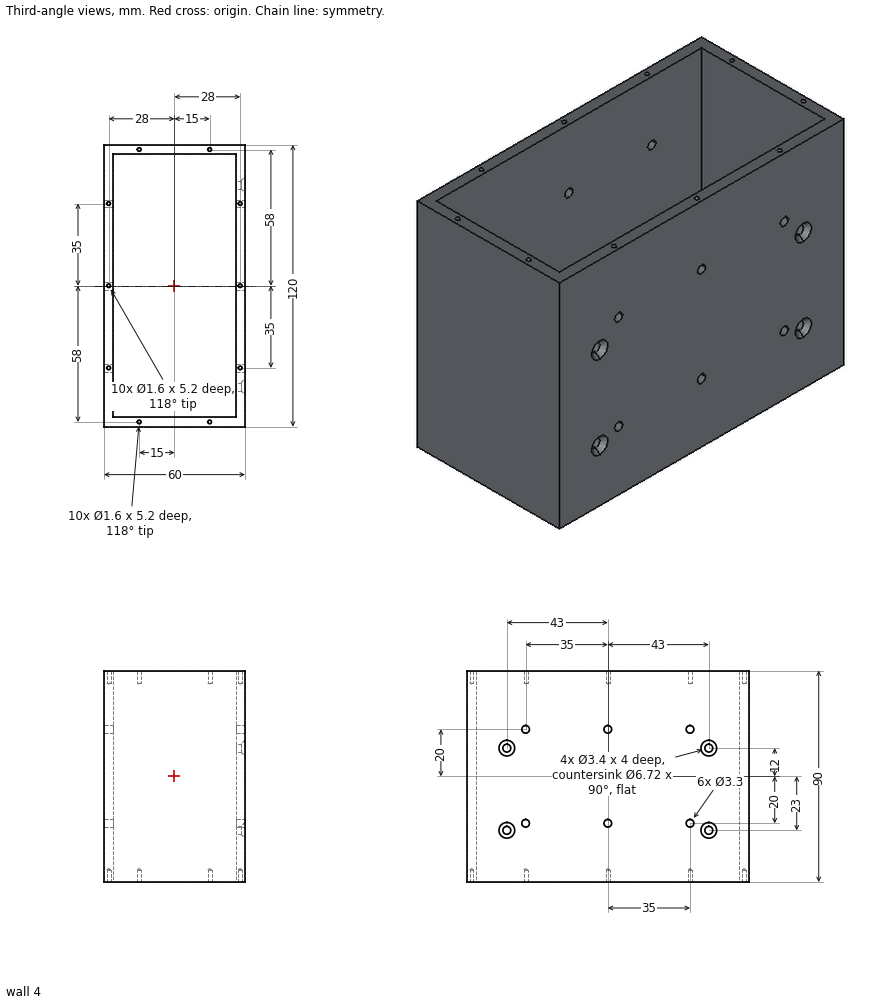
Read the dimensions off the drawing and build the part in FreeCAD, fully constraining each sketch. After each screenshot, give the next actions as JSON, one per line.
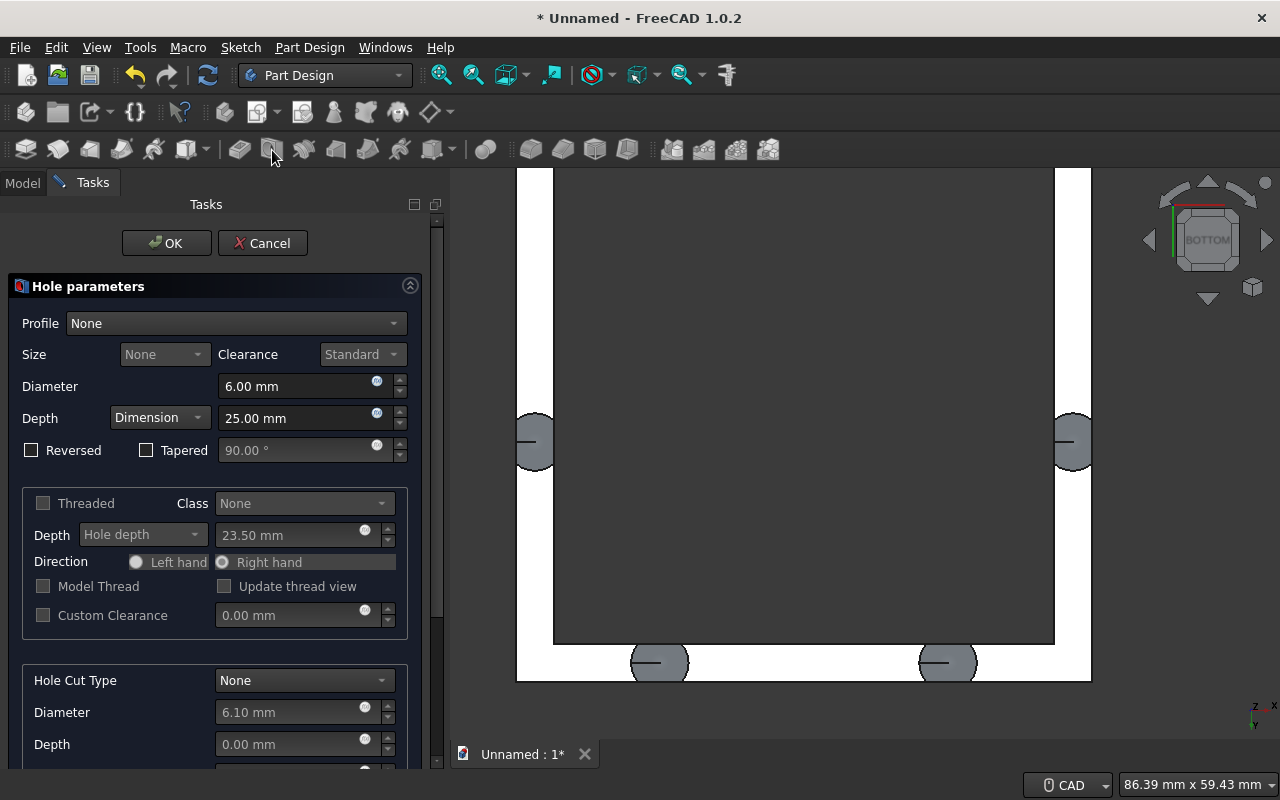
{"action": "triple_click", "coordinate": [305, 386]}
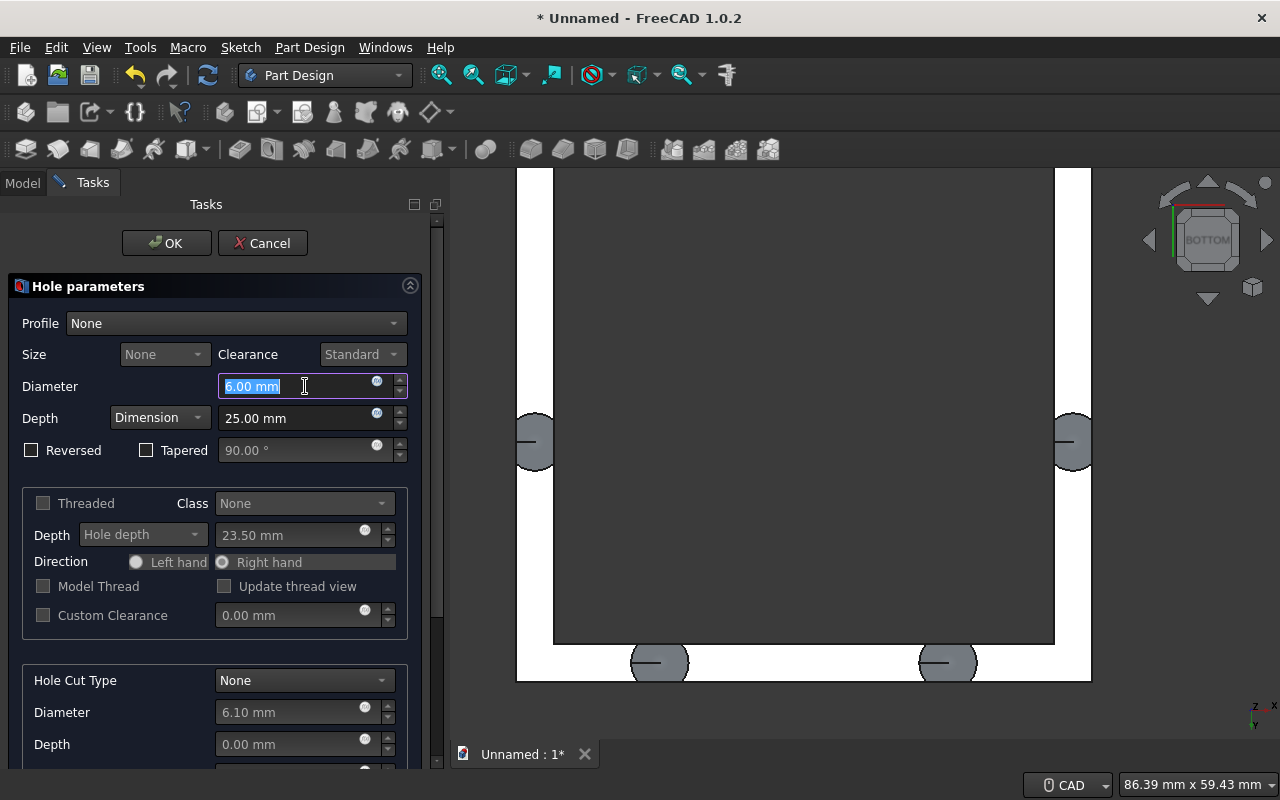
{"action": "type", "text": "1.6"}
{"action": "key", "text": "Tab"}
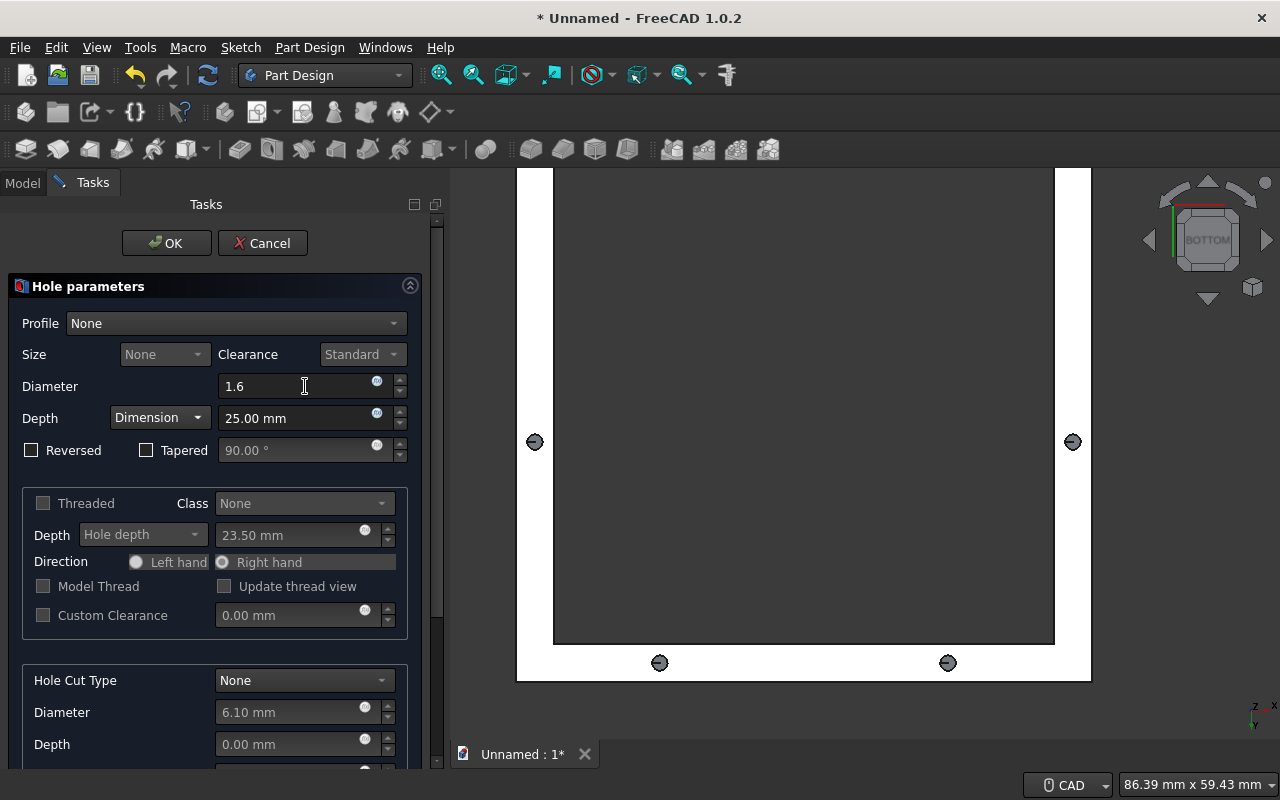
{"action": "triple_click", "coordinate": [305, 418]}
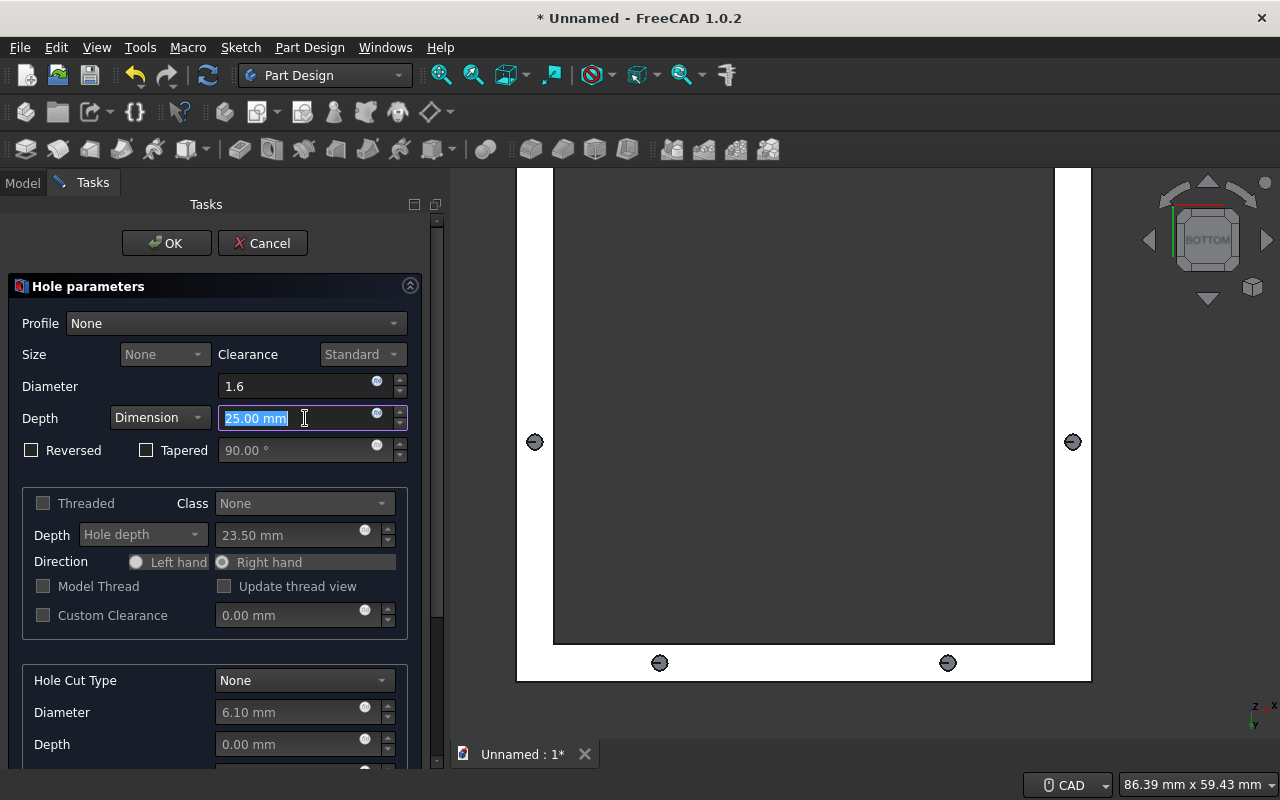
{"action": "type", "text": "5.2"}
{"action": "key", "text": "Tab"}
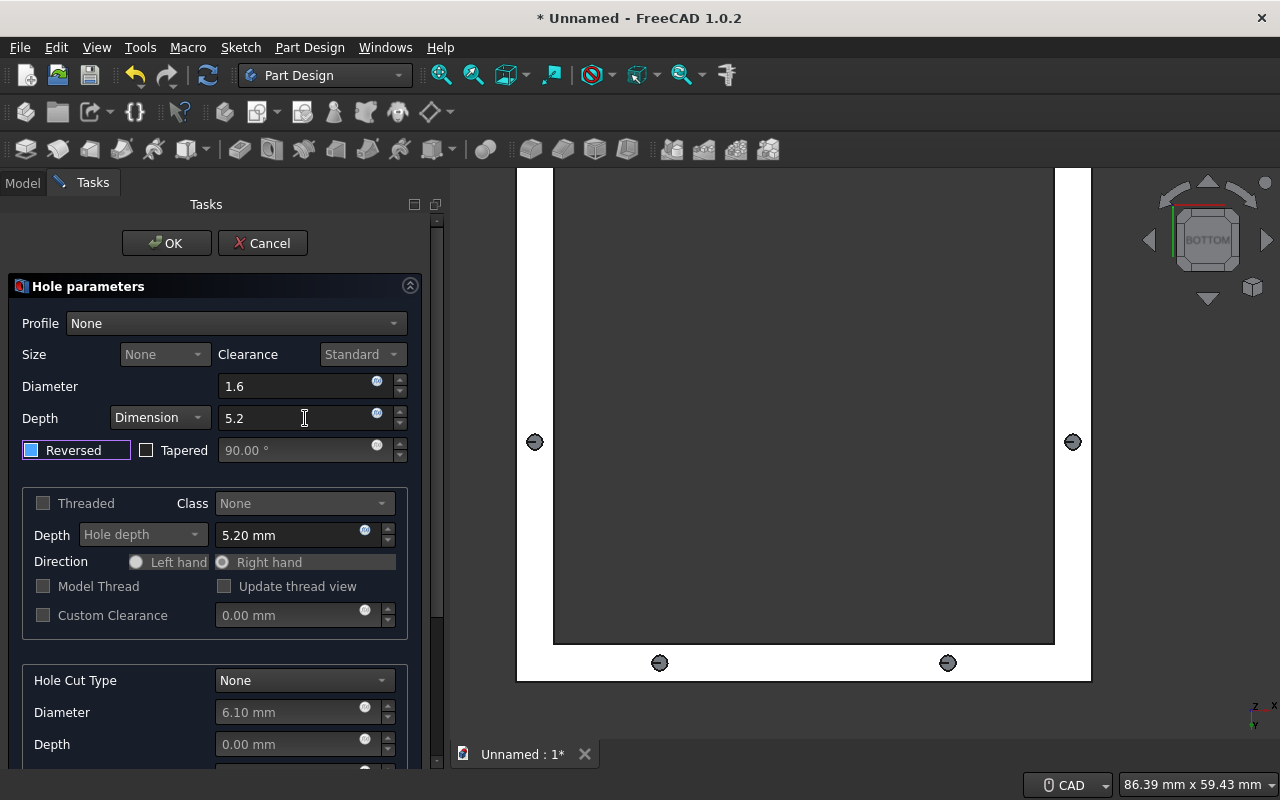
{"action": "left_click", "coordinate": [167, 243]}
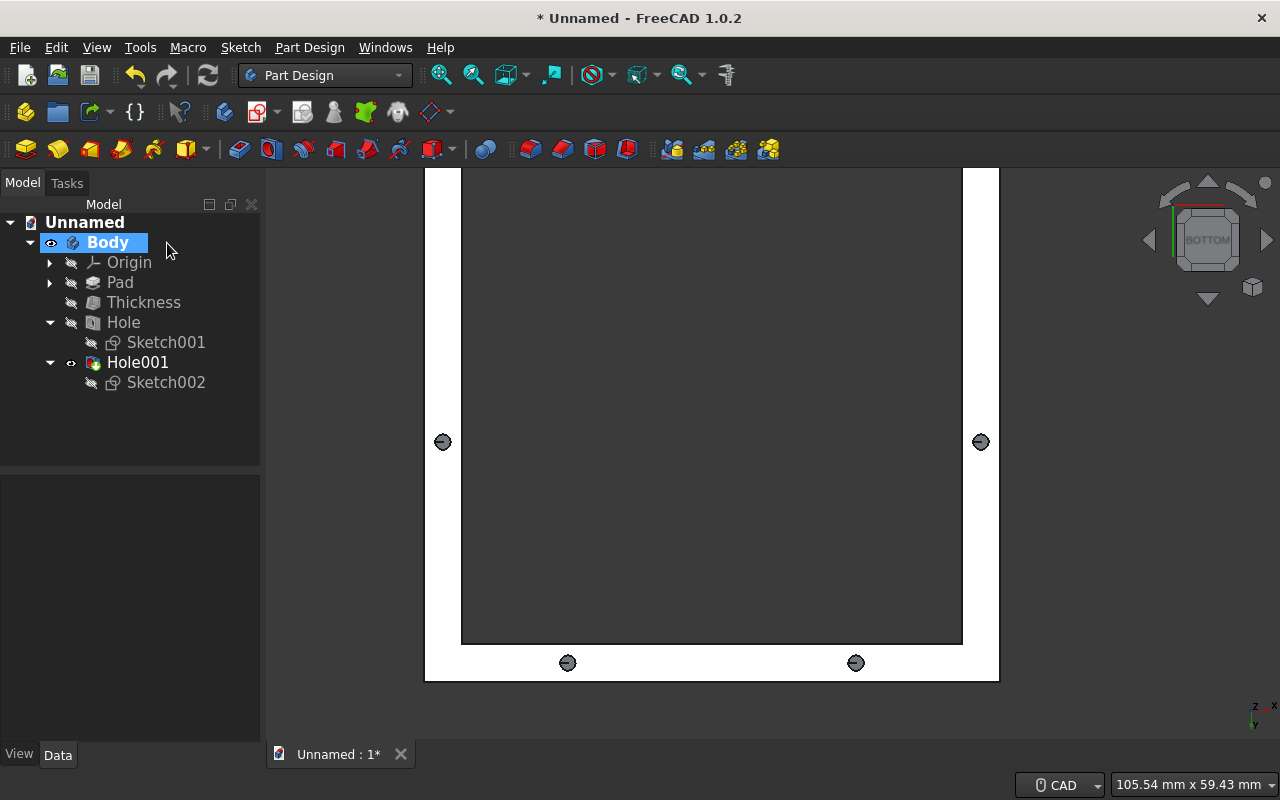
{"action": "left_click", "coordinate": [442, 76]}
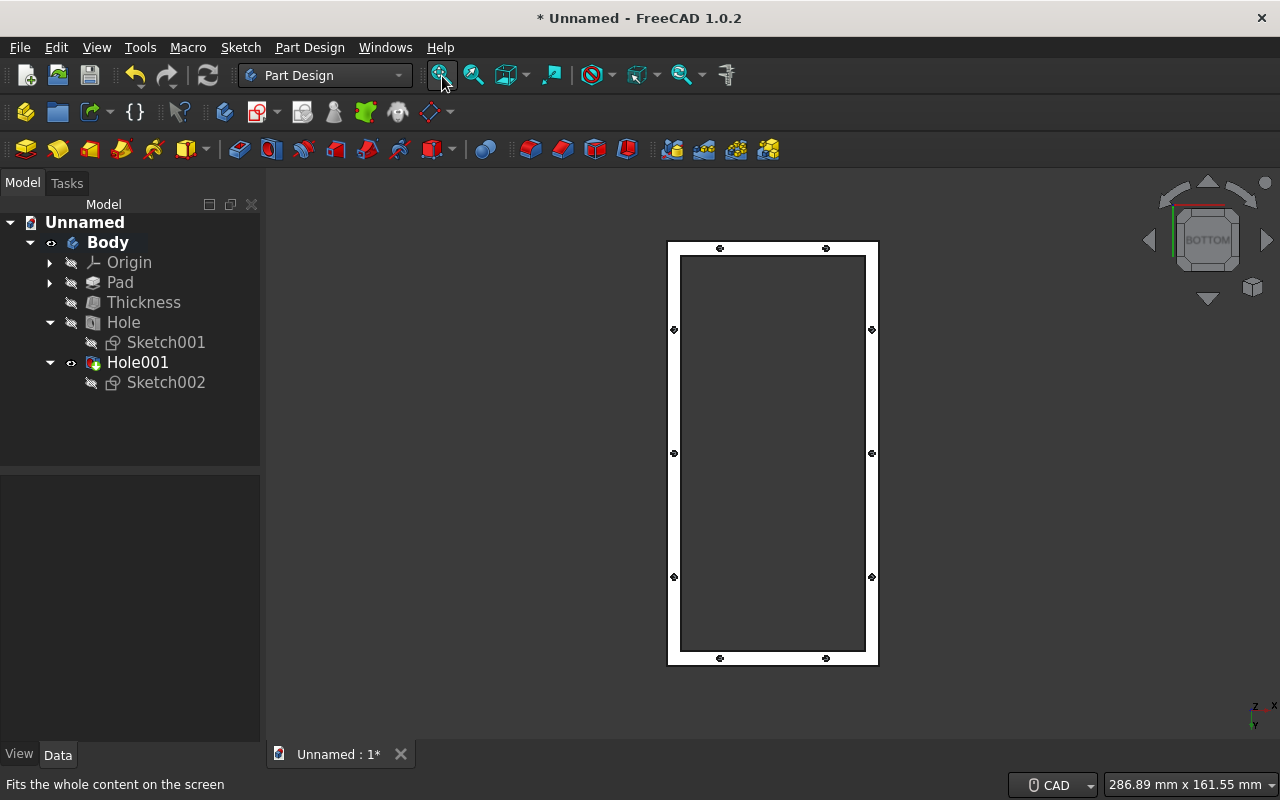
{"action": "key", "text": "0"}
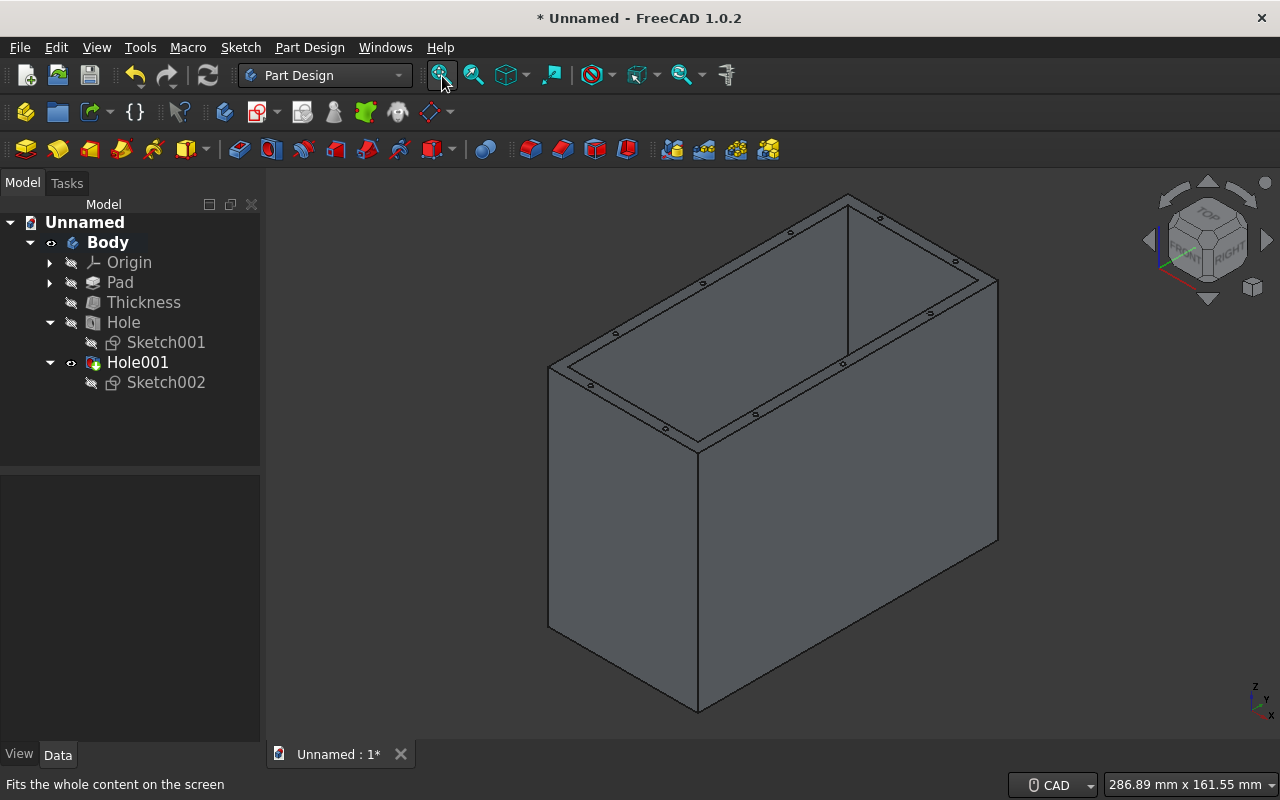
{"action": "left_click", "coordinate": [848, 496]}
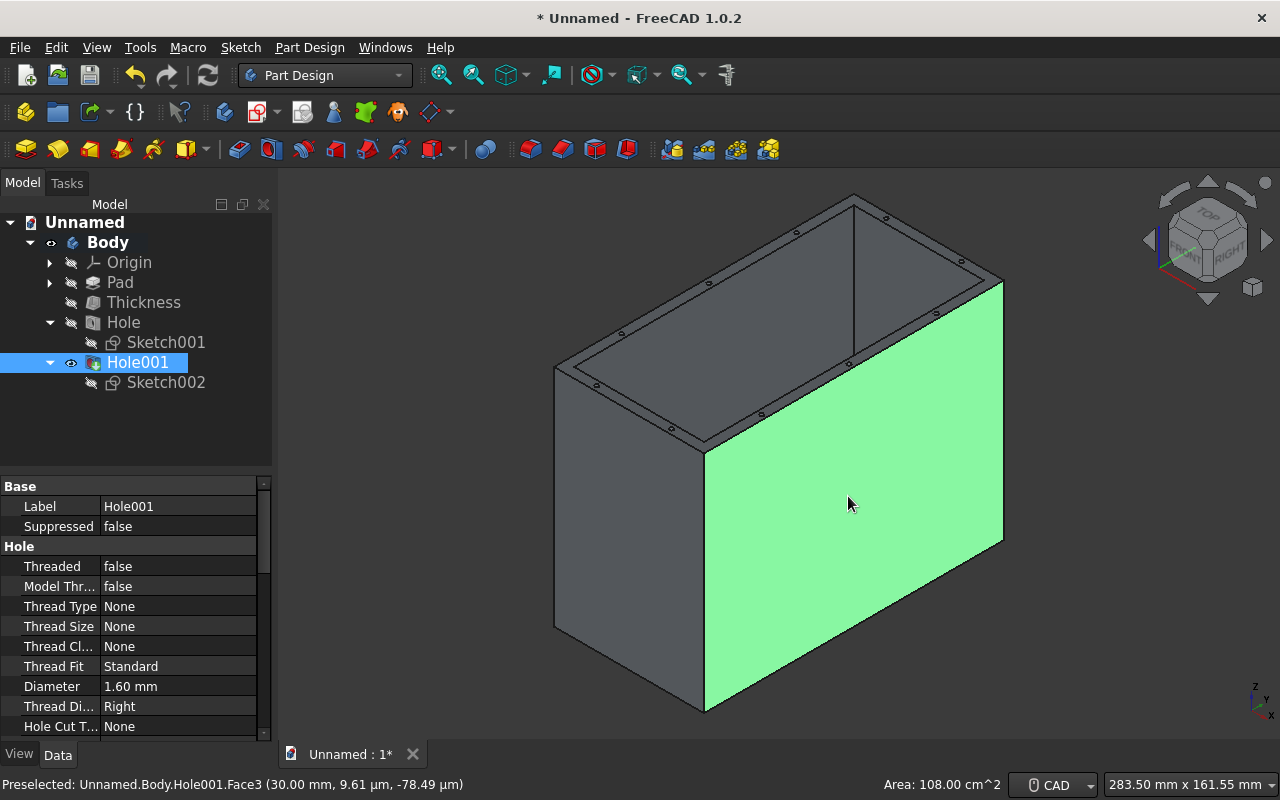
{"action": "left_click", "coordinate": [258, 112]}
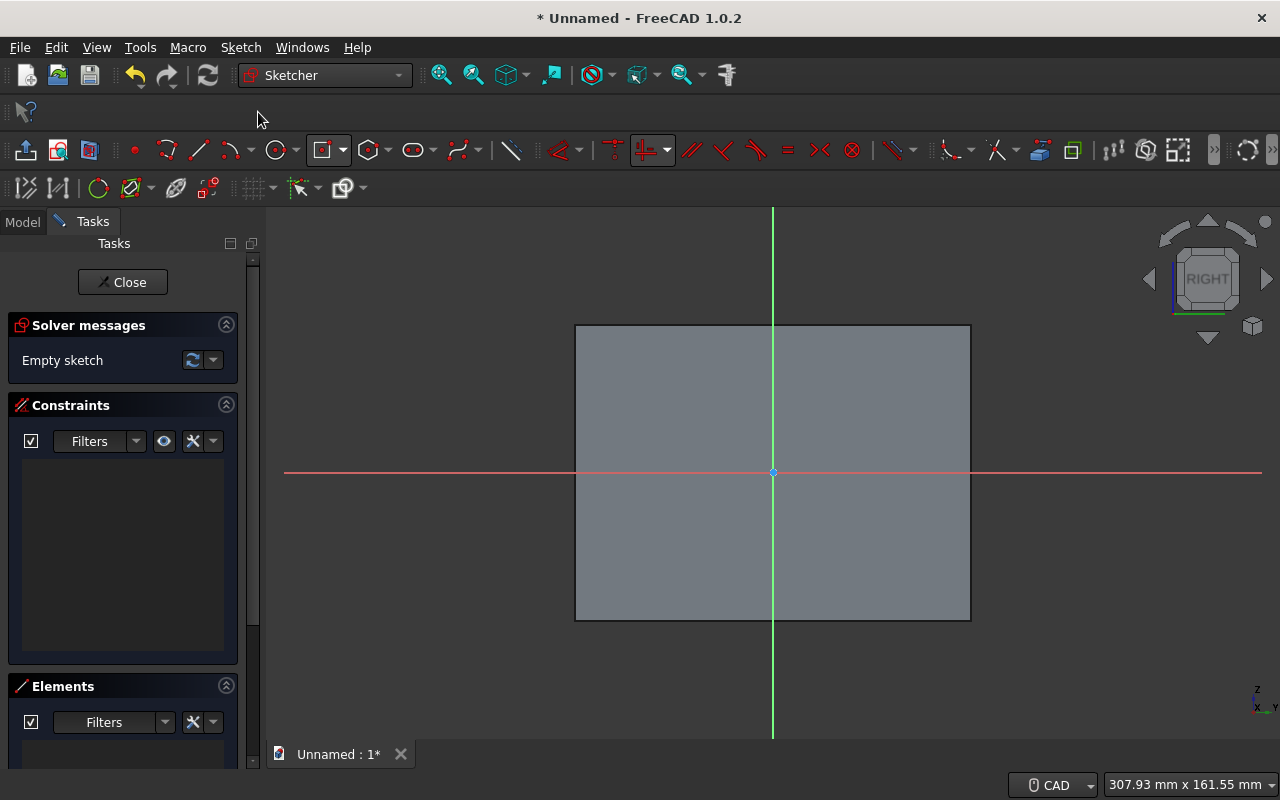
{"action": "scroll", "coordinate": [856, 513], "scroll_direction": "up", "scroll_amount": 3}